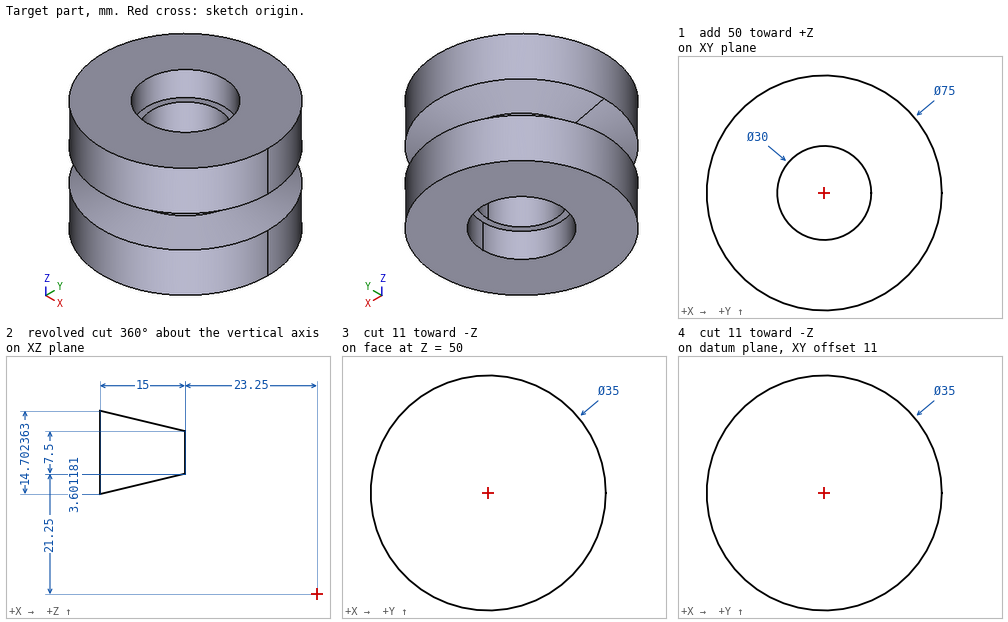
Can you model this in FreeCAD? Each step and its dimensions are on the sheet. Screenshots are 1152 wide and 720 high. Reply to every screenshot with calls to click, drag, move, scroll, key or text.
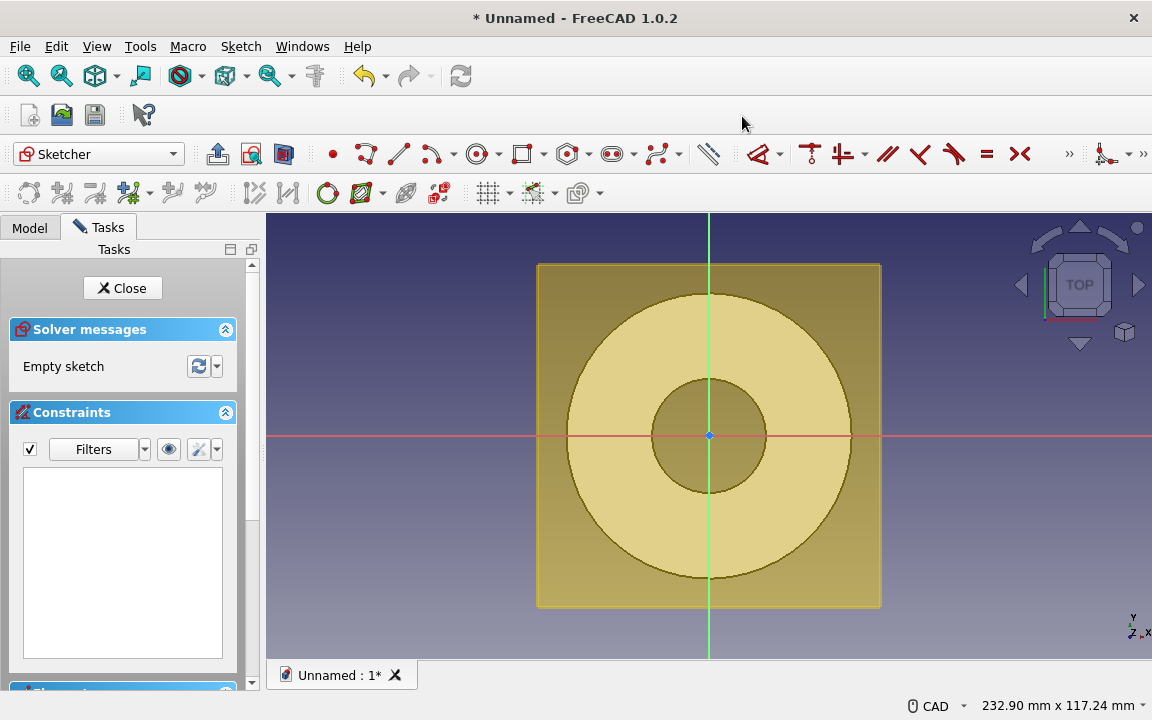
scroll(765, 436, up, 4)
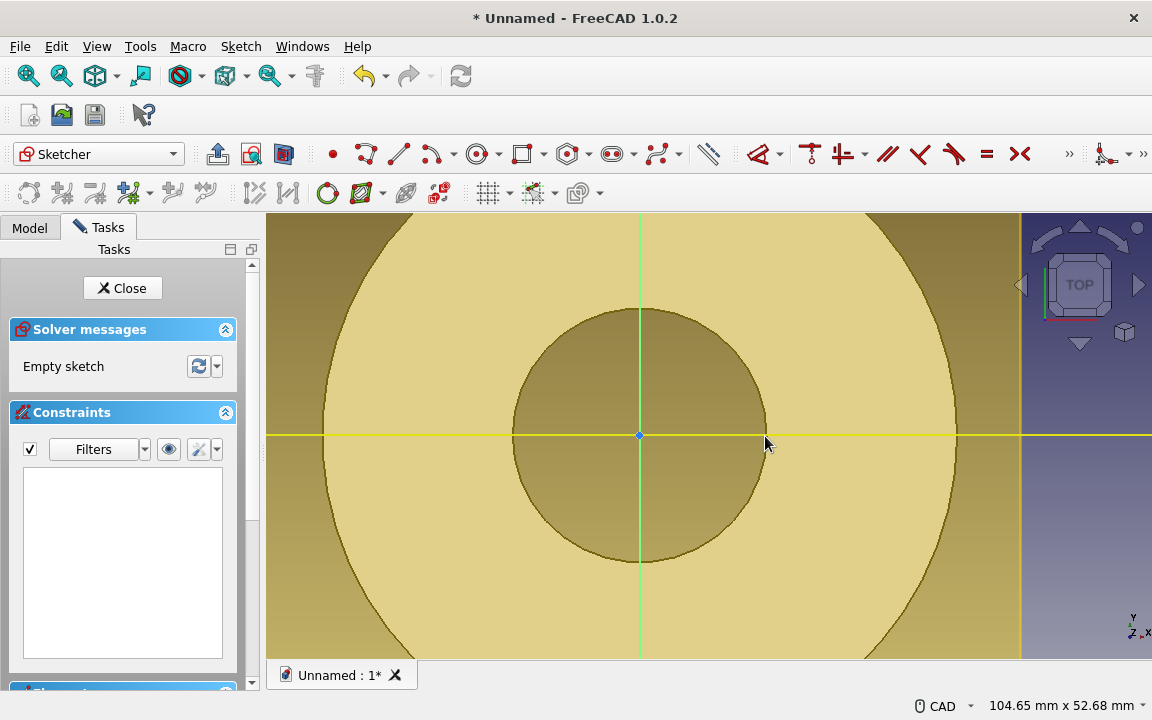
key(g)
key(c)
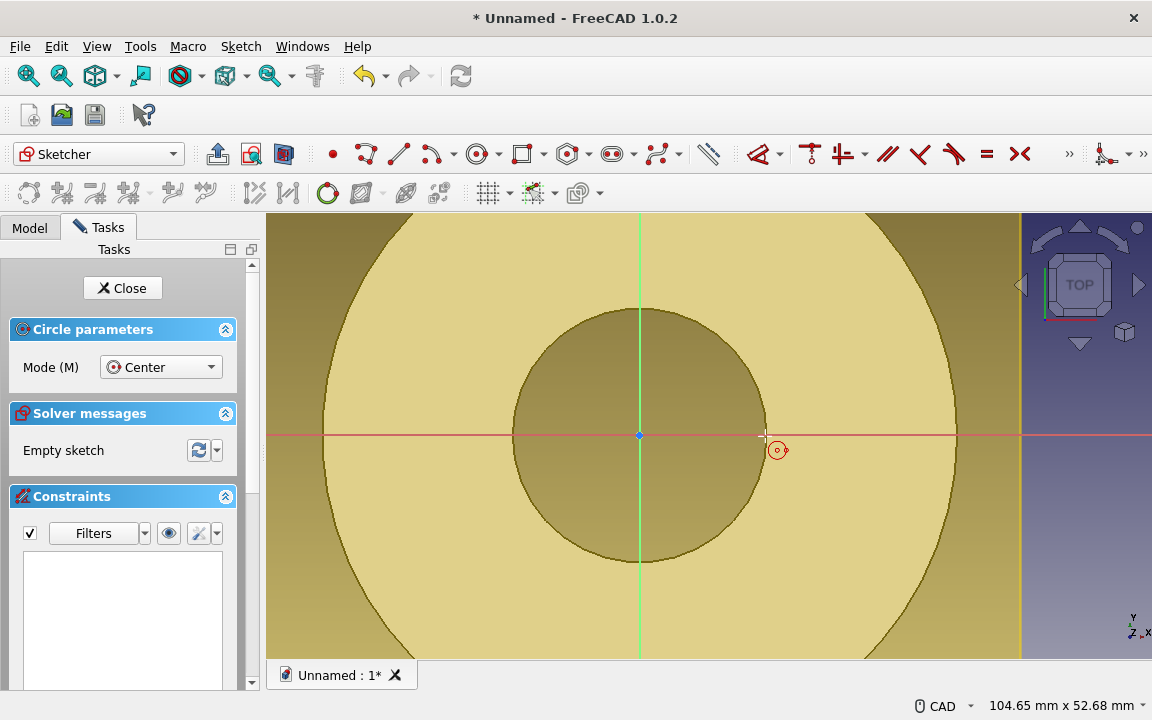
click(640, 435)
move(744, 331)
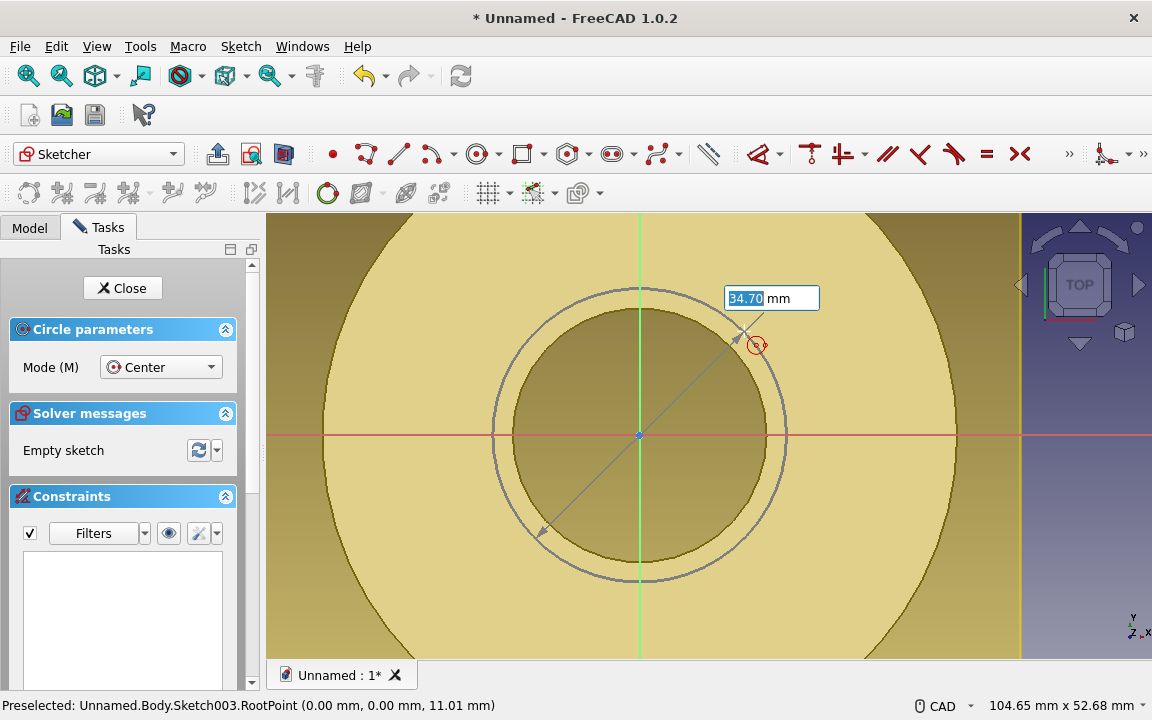
text(35)
key(Return)
key(Escape)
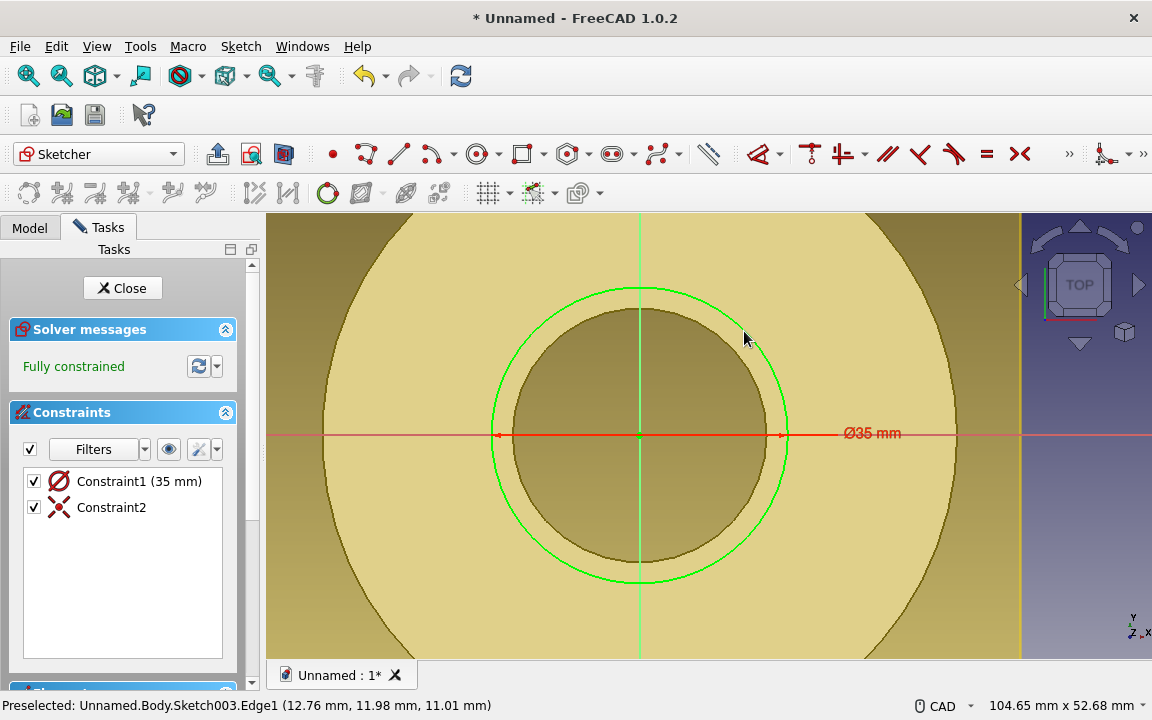
click(123, 288)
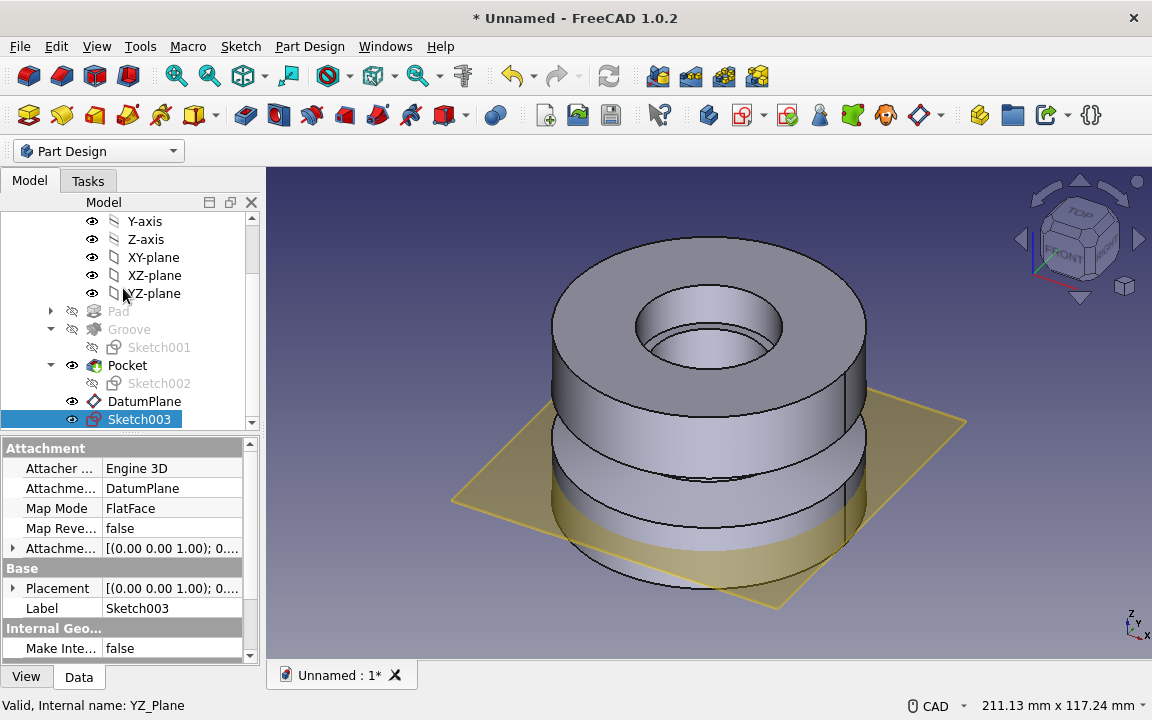
click(246, 116)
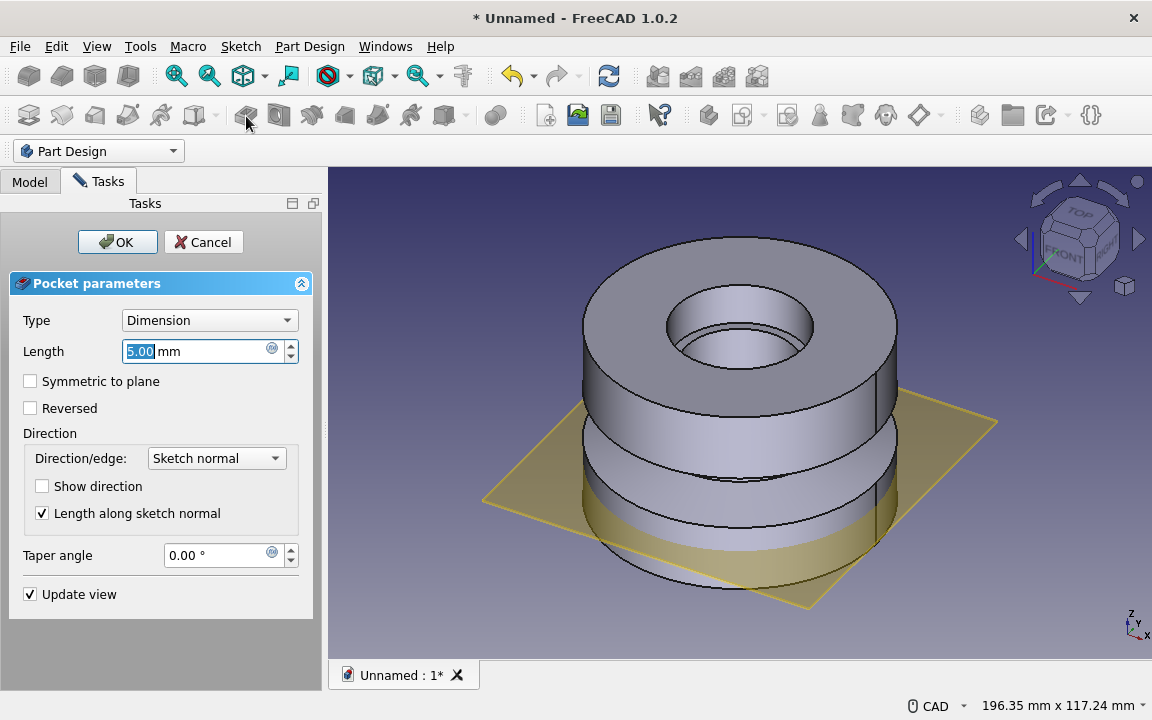
text(11)
key(Tab)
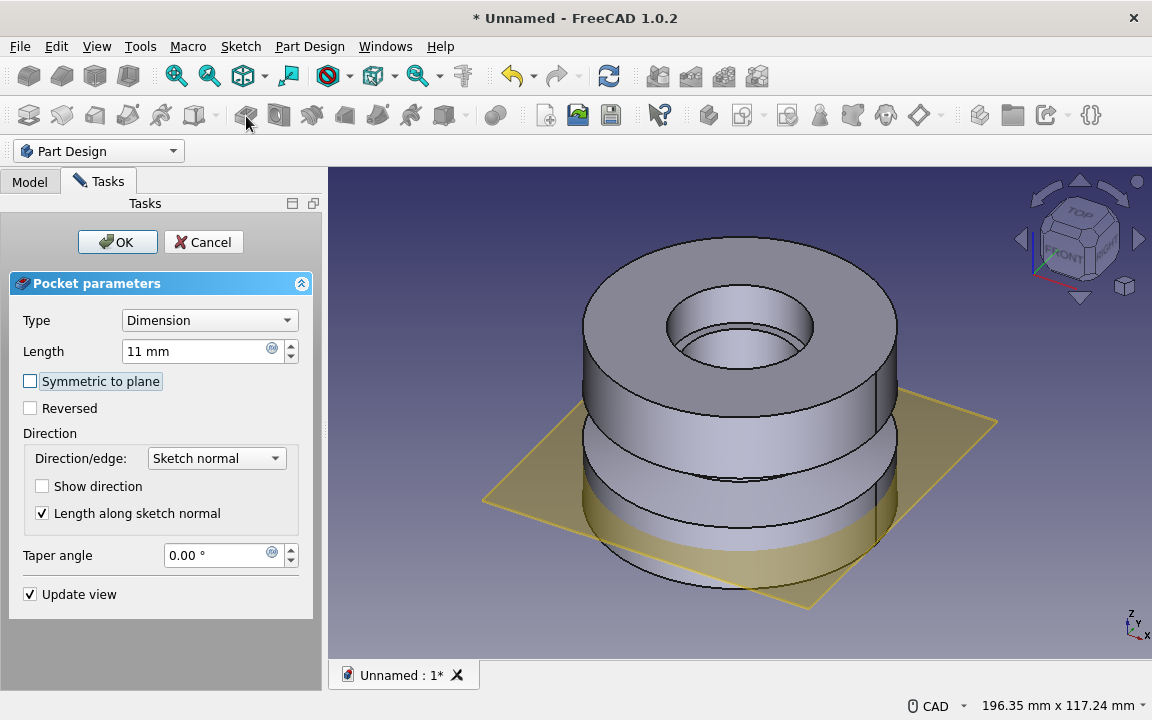
click(118, 242)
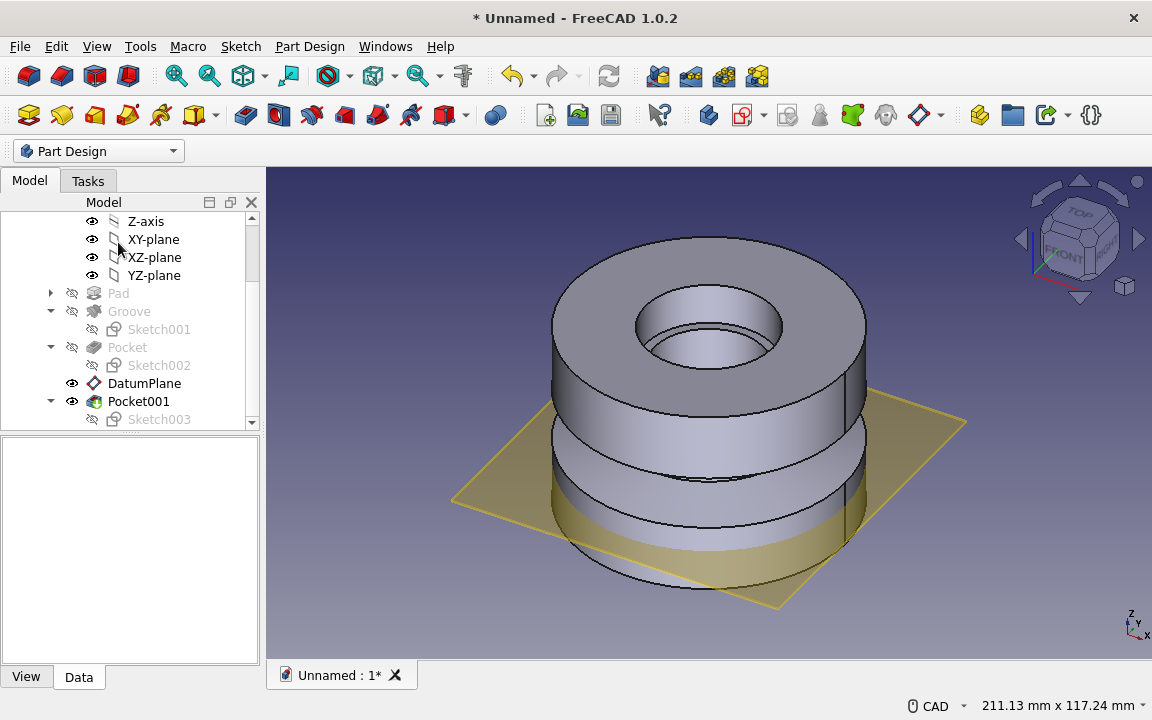
click(117, 383)
key(space)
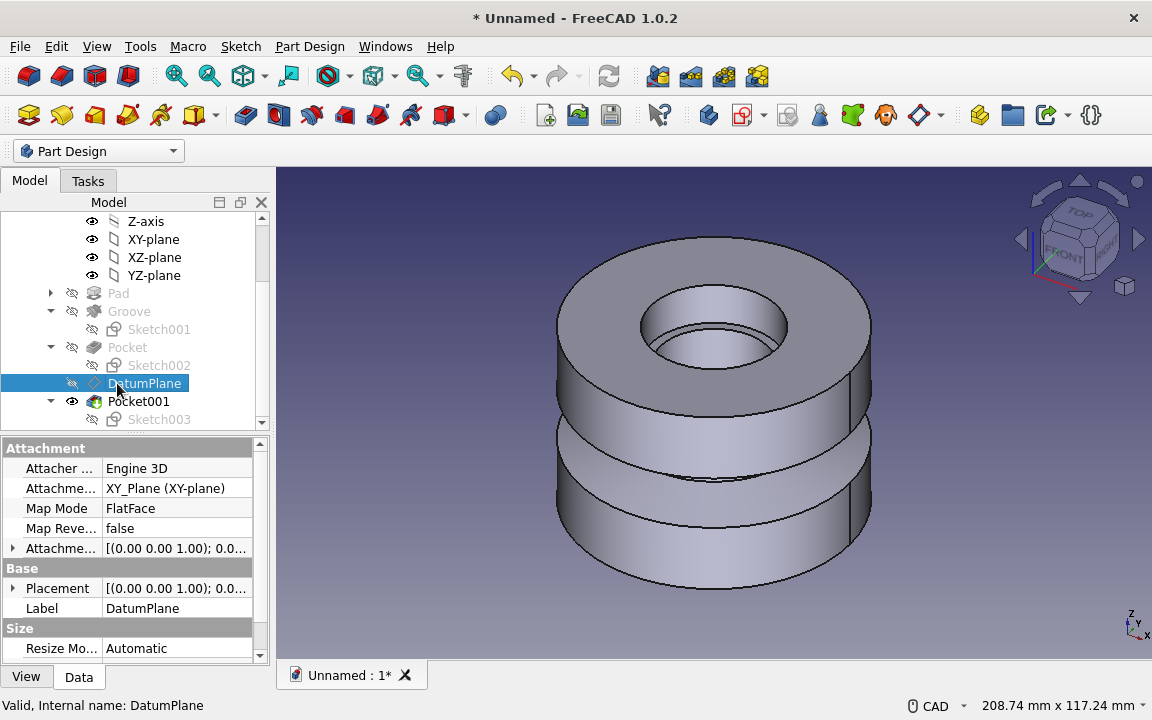
key(0)